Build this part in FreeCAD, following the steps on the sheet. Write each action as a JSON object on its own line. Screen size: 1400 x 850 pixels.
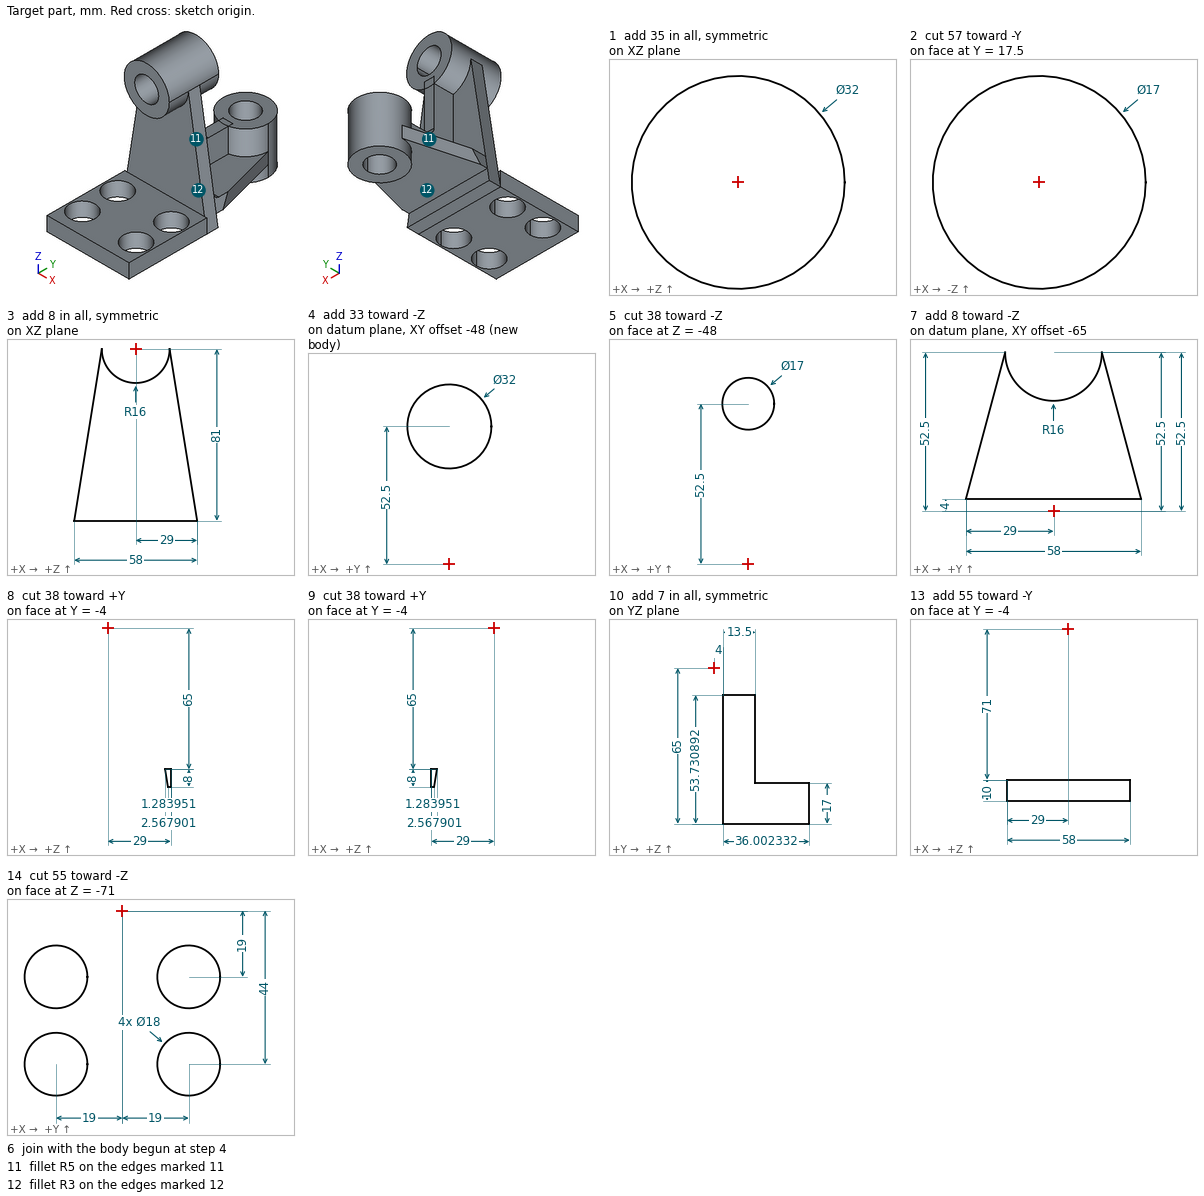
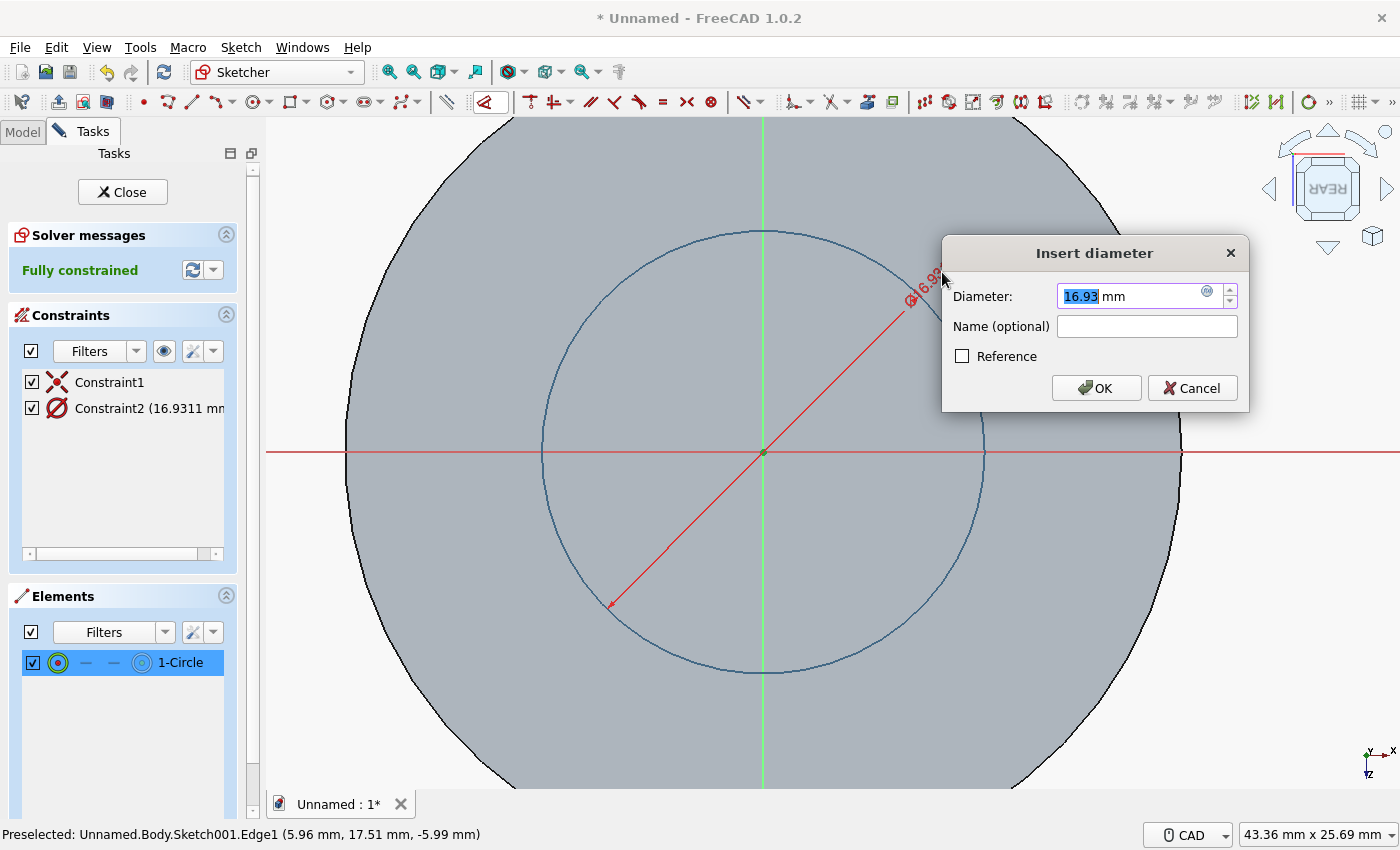
{"action": "type", "text": "17"}
{"action": "key", "text": "Return"}
{"action": "key", "text": "Escape"}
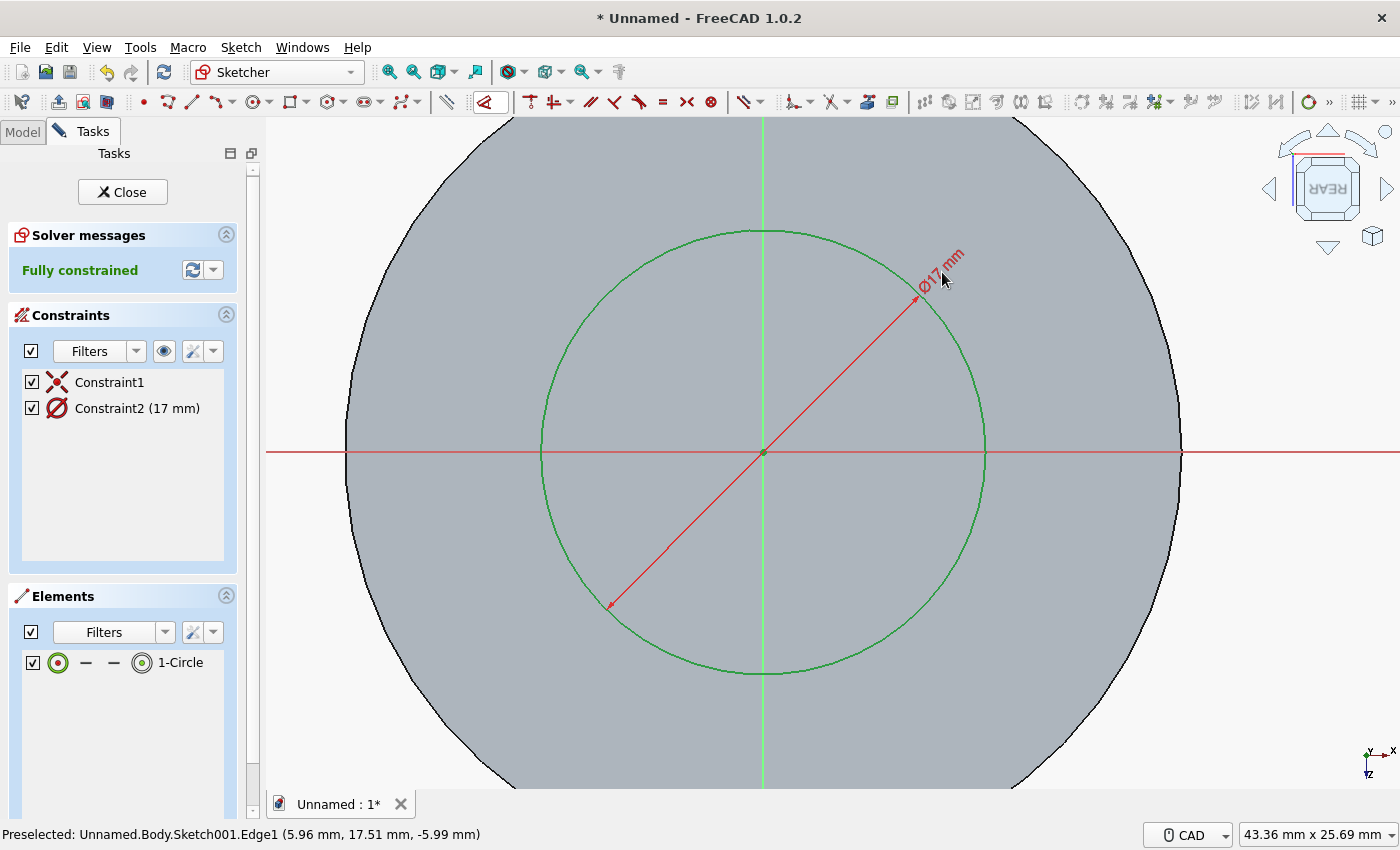
{"action": "left_click", "coordinate": [123, 192]}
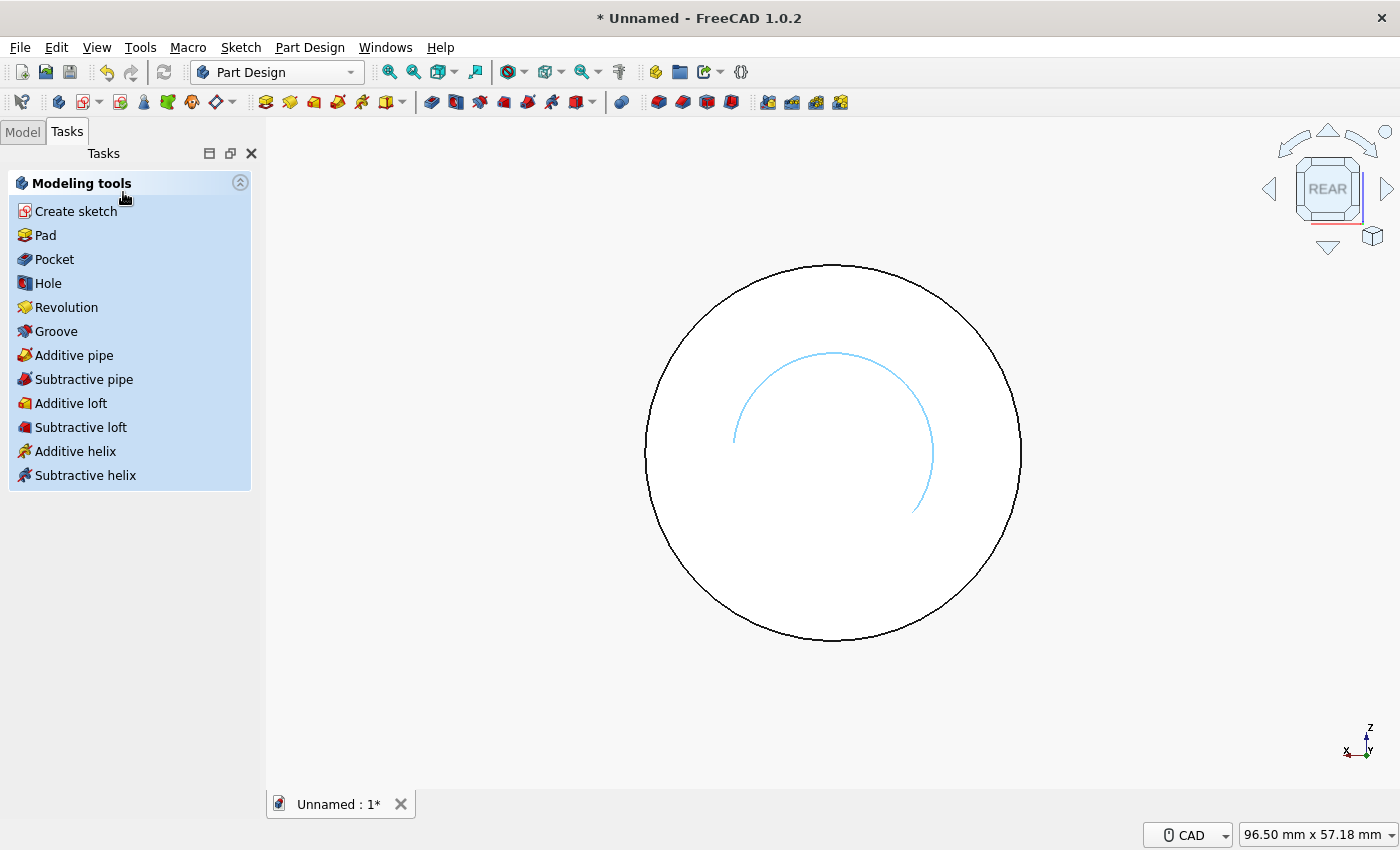
{"action": "left_click", "coordinate": [432, 102]}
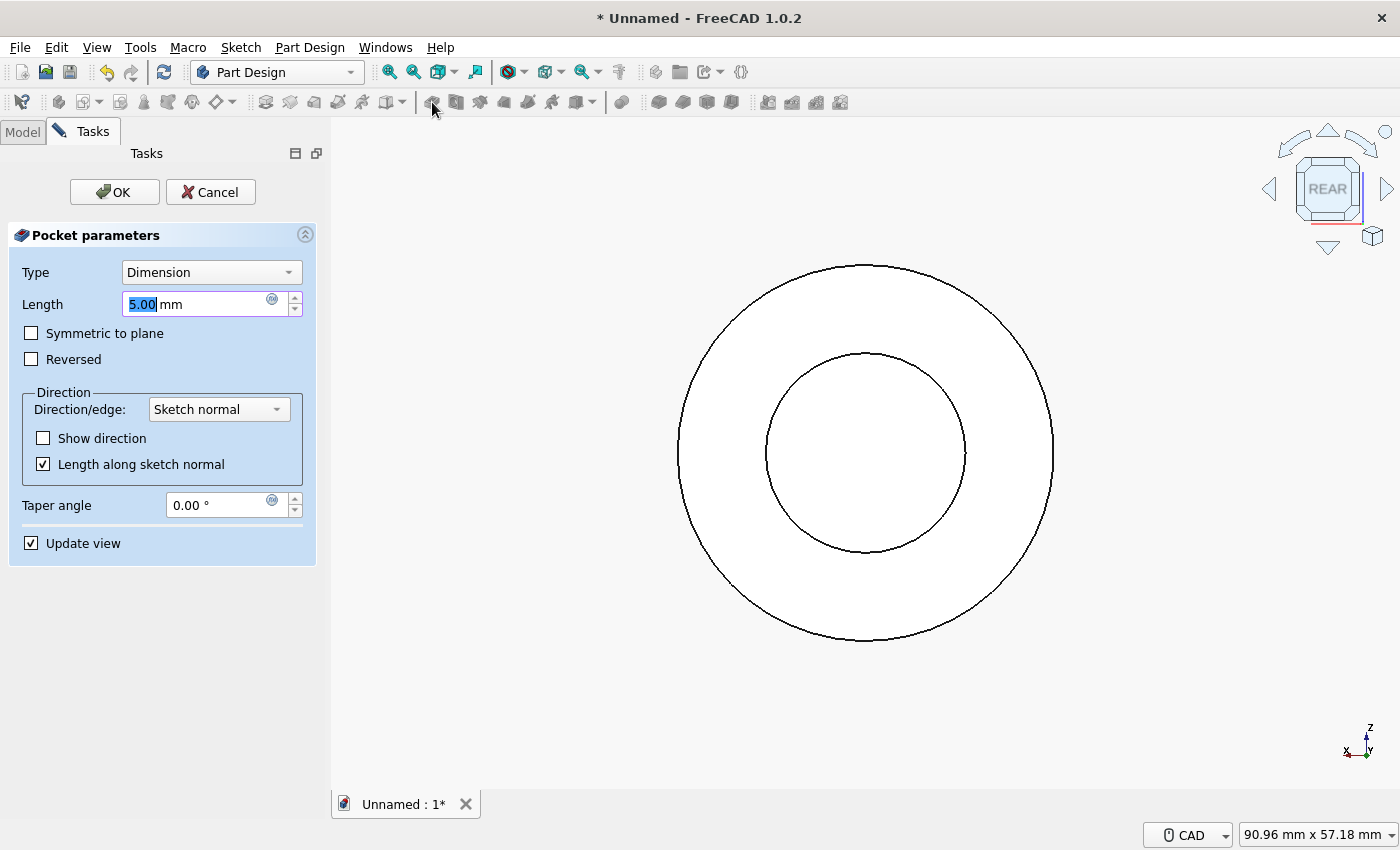
{"action": "type", "text": "57"}
{"action": "key", "text": "Tab"}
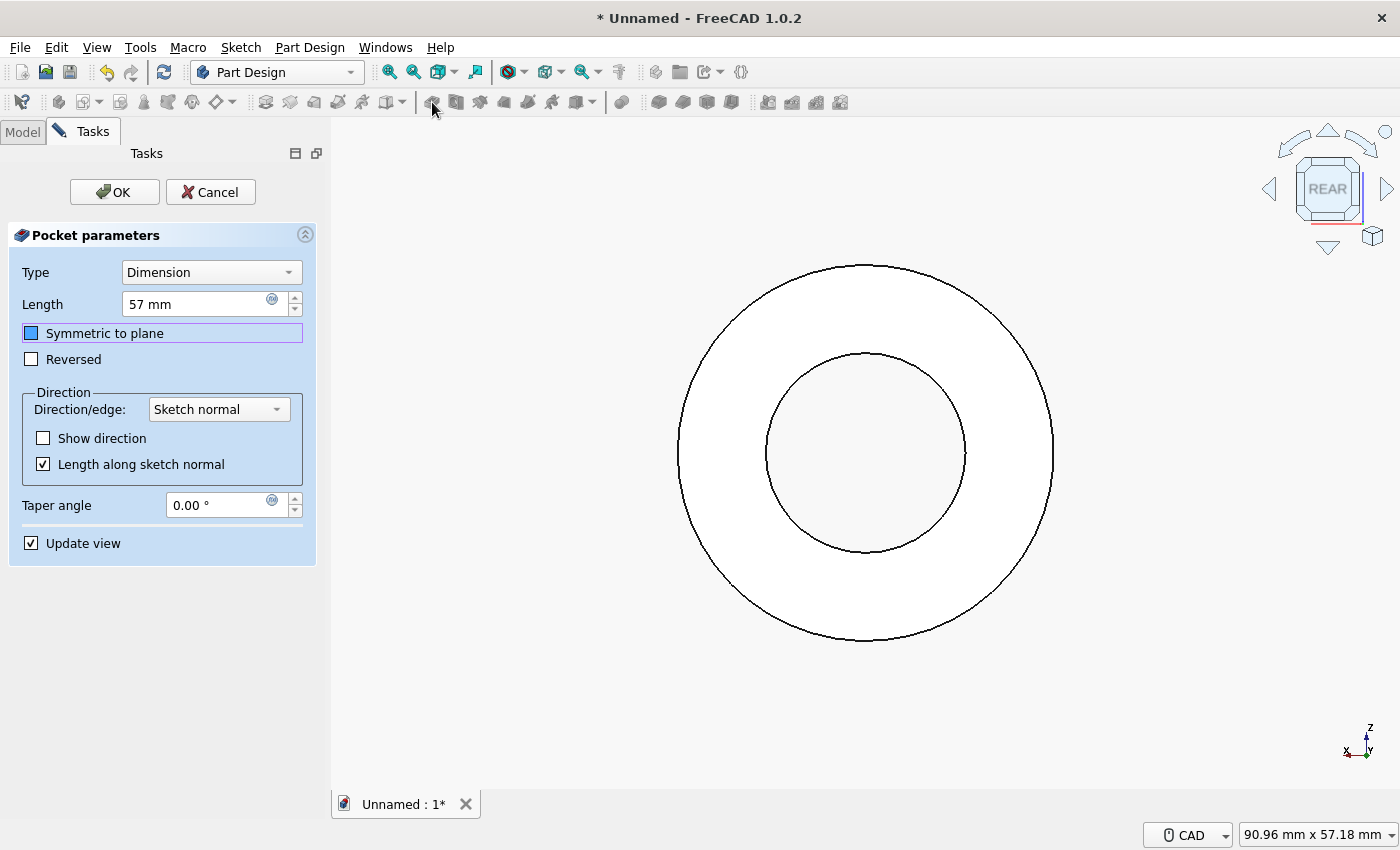
{"action": "left_click", "coordinate": [115, 192]}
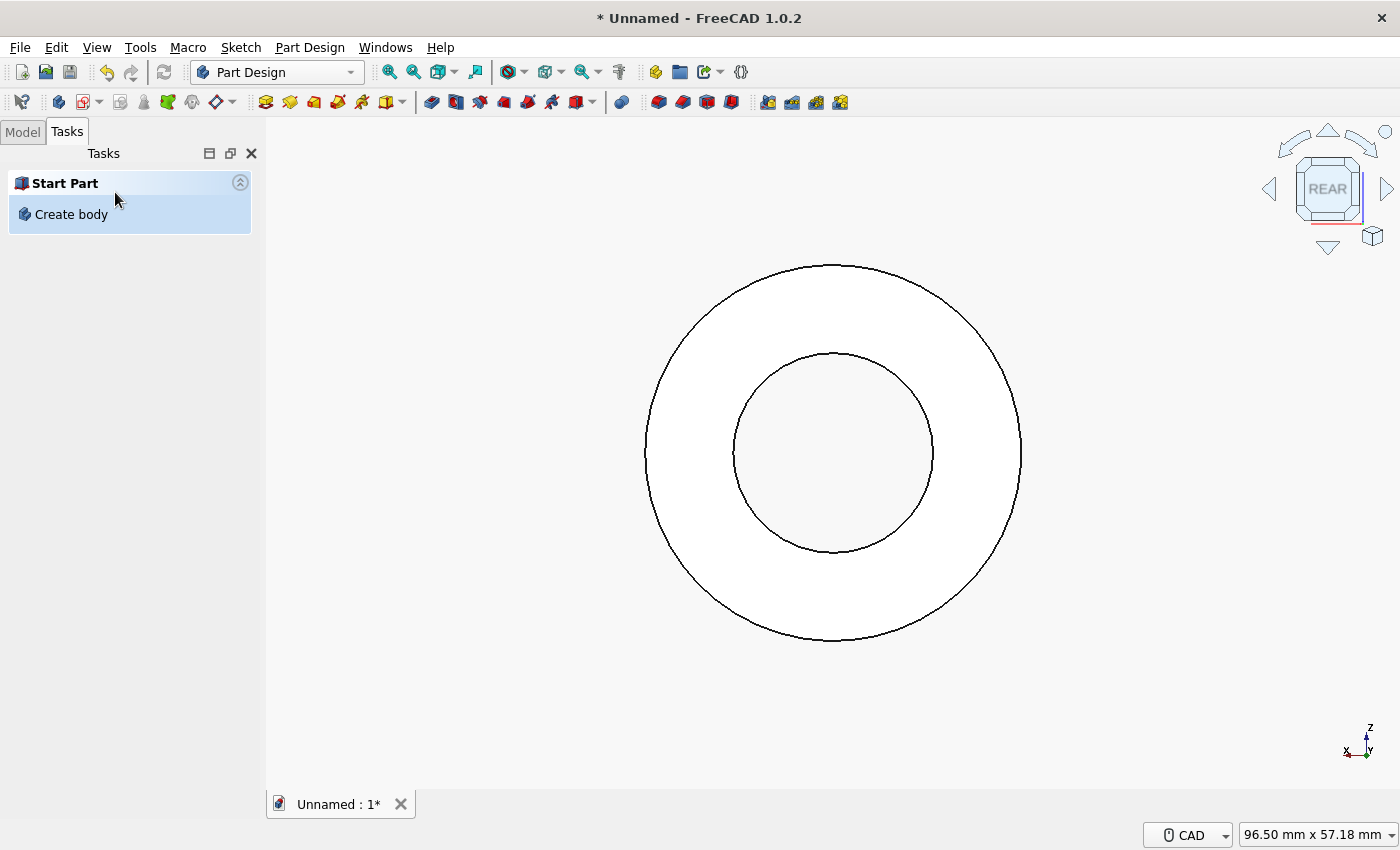
{"action": "left_click", "coordinate": [84, 102]}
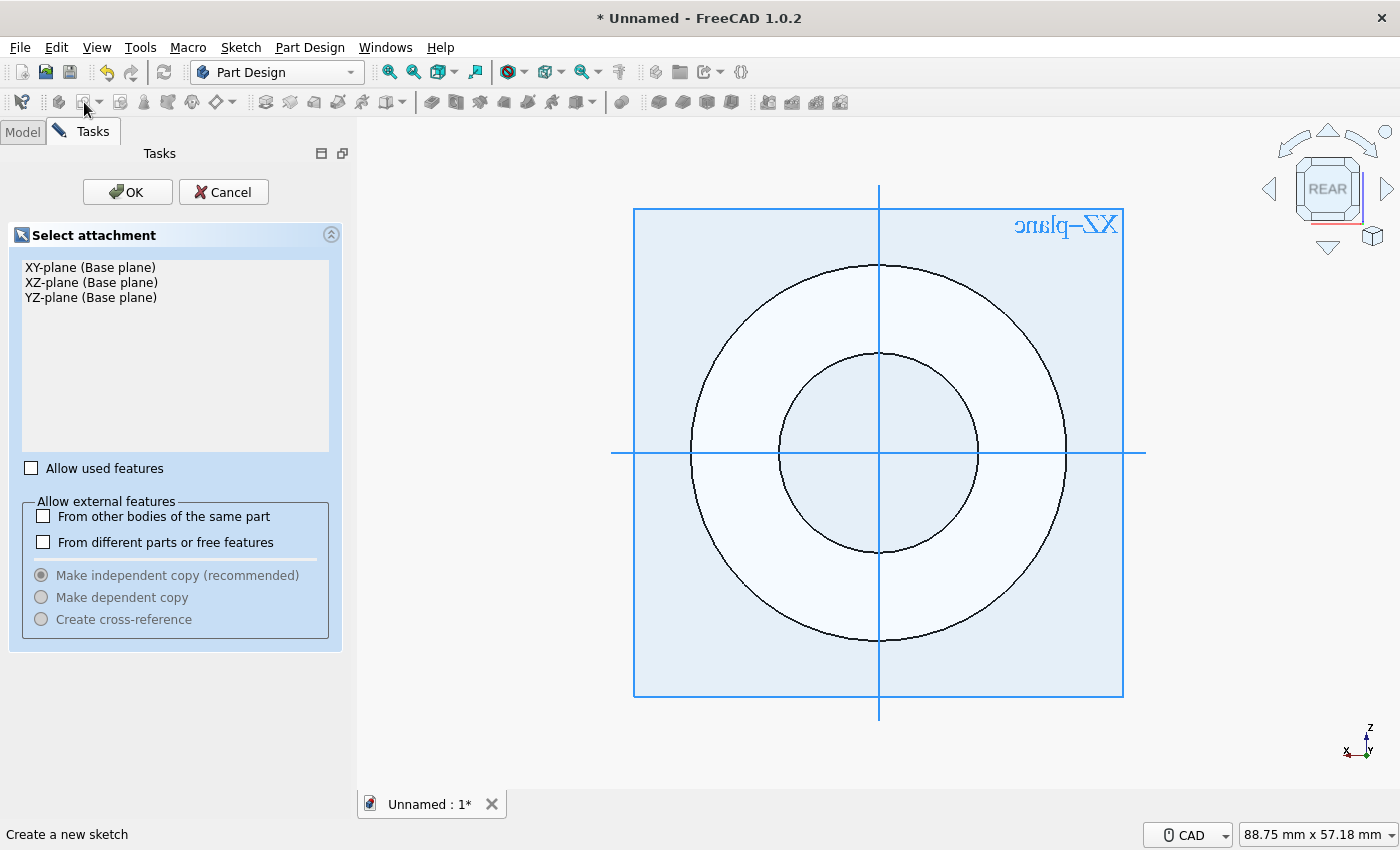
{"action": "left_click", "coordinate": [82, 282]}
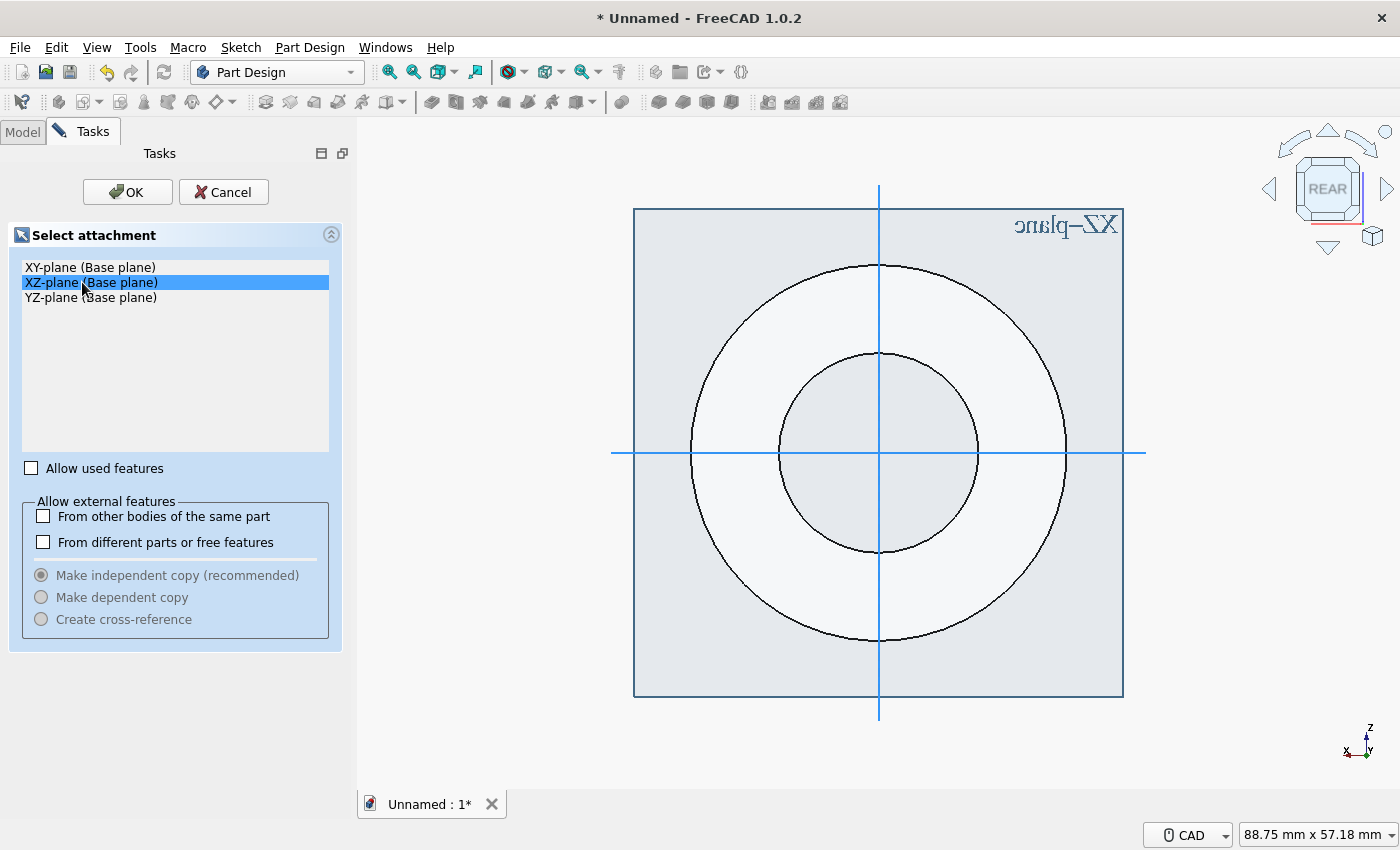
{"action": "left_click", "coordinate": [128, 192]}